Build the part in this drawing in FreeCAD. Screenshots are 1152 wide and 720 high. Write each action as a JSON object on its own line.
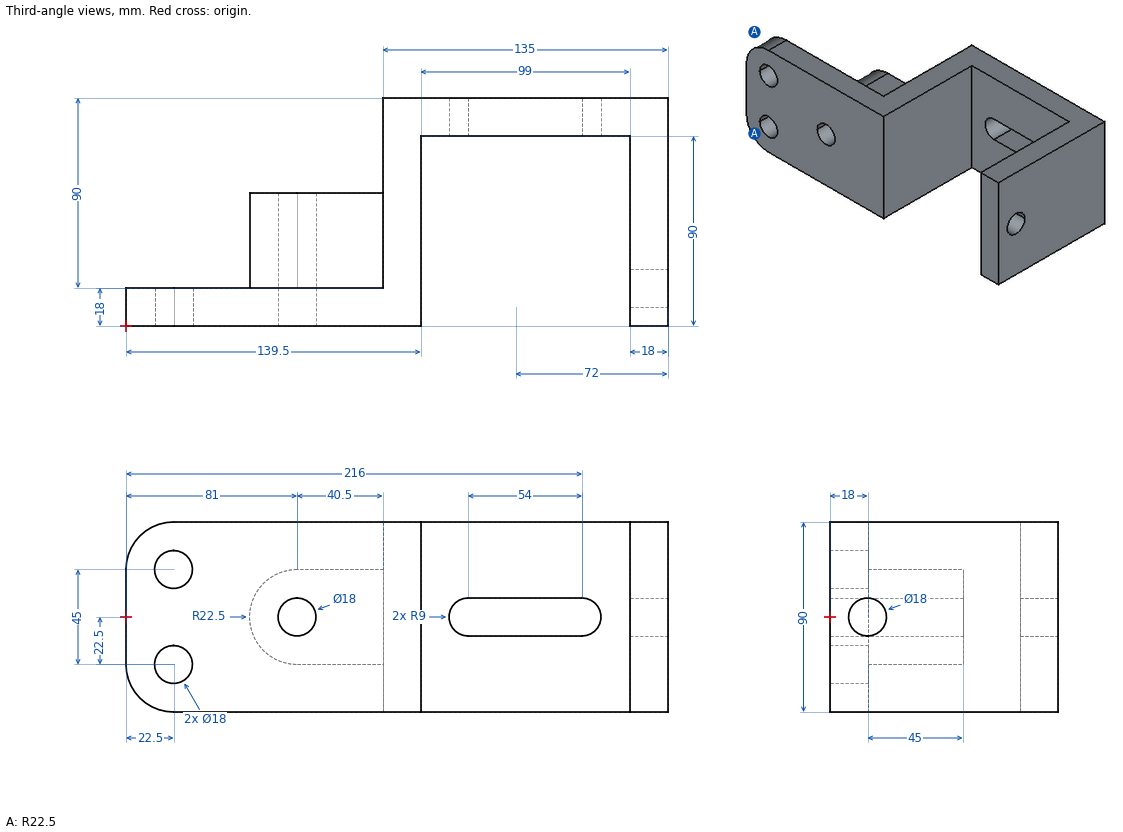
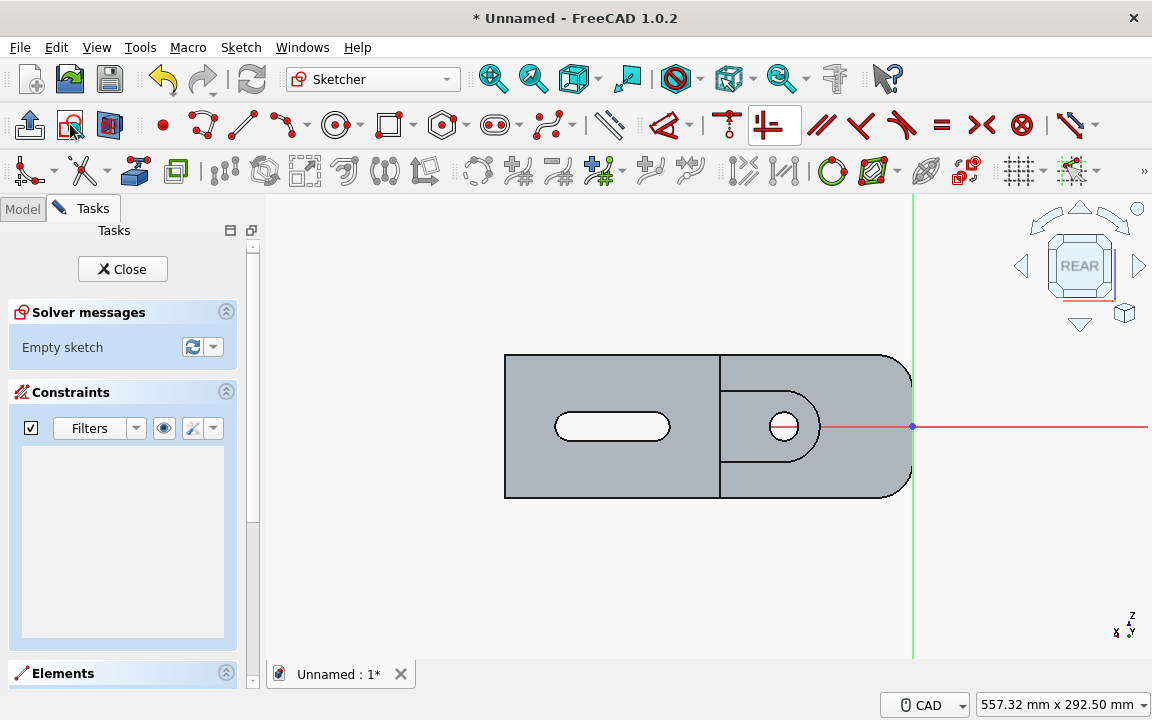
{"action": "left_click", "coordinate": [110, 126]}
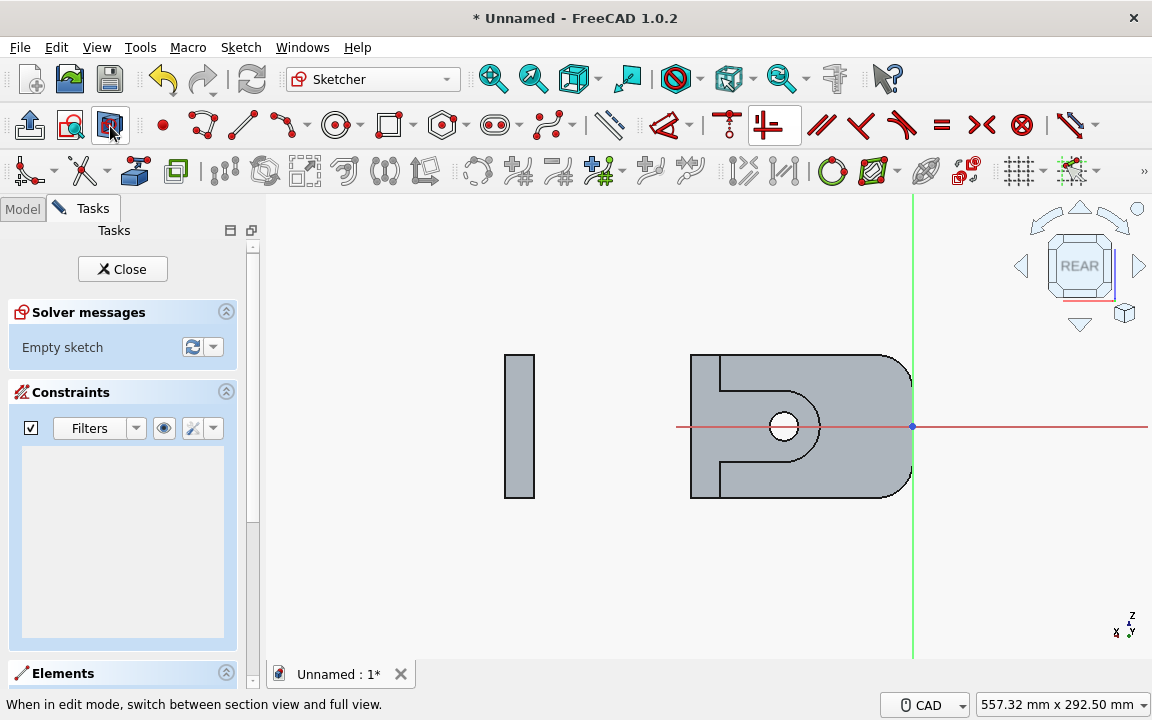
{"action": "scroll", "coordinate": [987, 426], "scroll_direction": "up", "scroll_amount": 5}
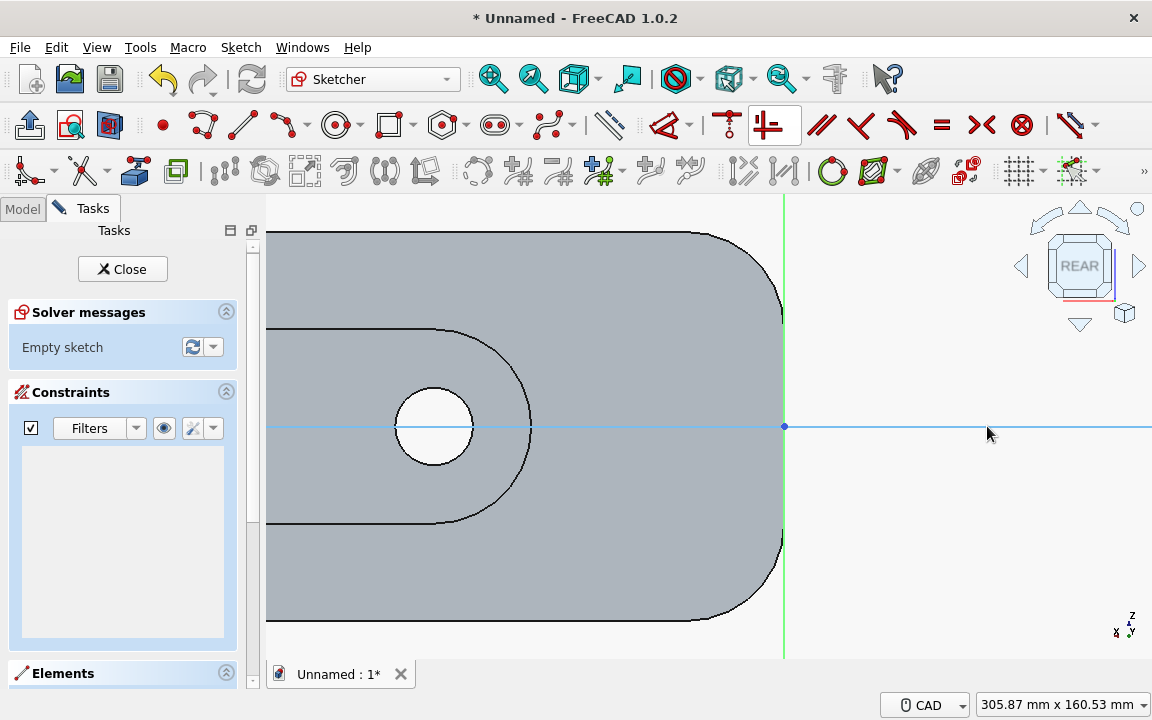
{"action": "left_click", "coordinate": [336, 126]}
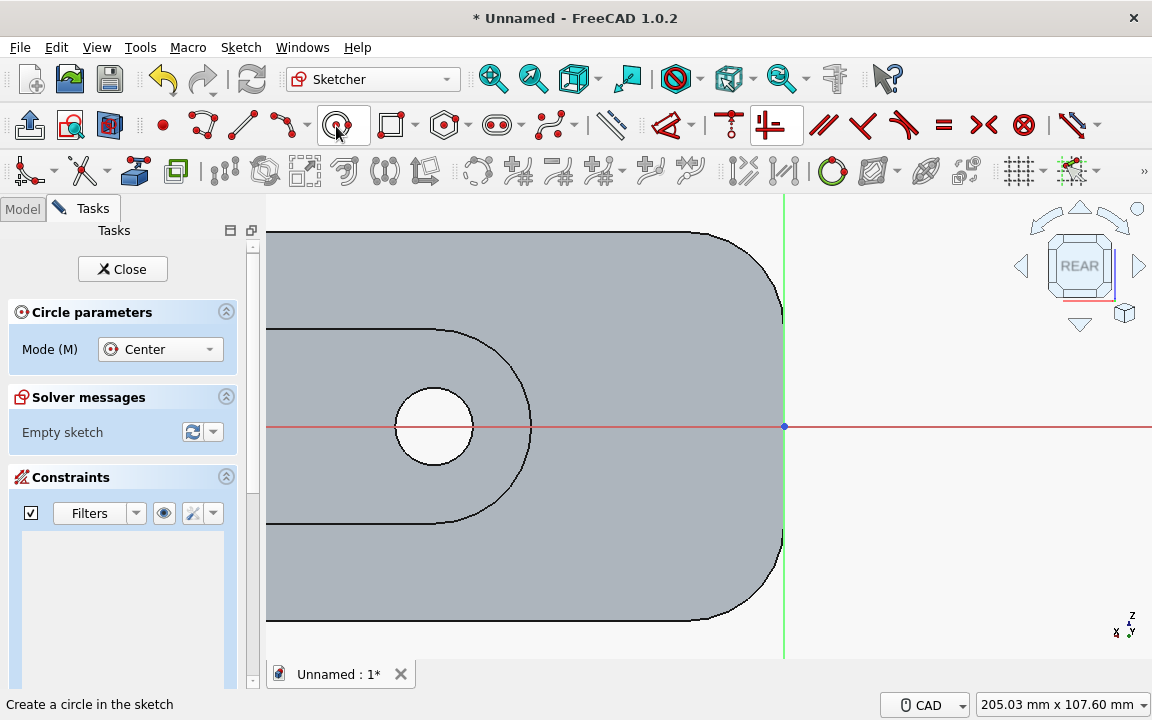
{"action": "left_click", "coordinate": [687, 524]}
{"action": "mouse_move", "coordinate": [714, 496]}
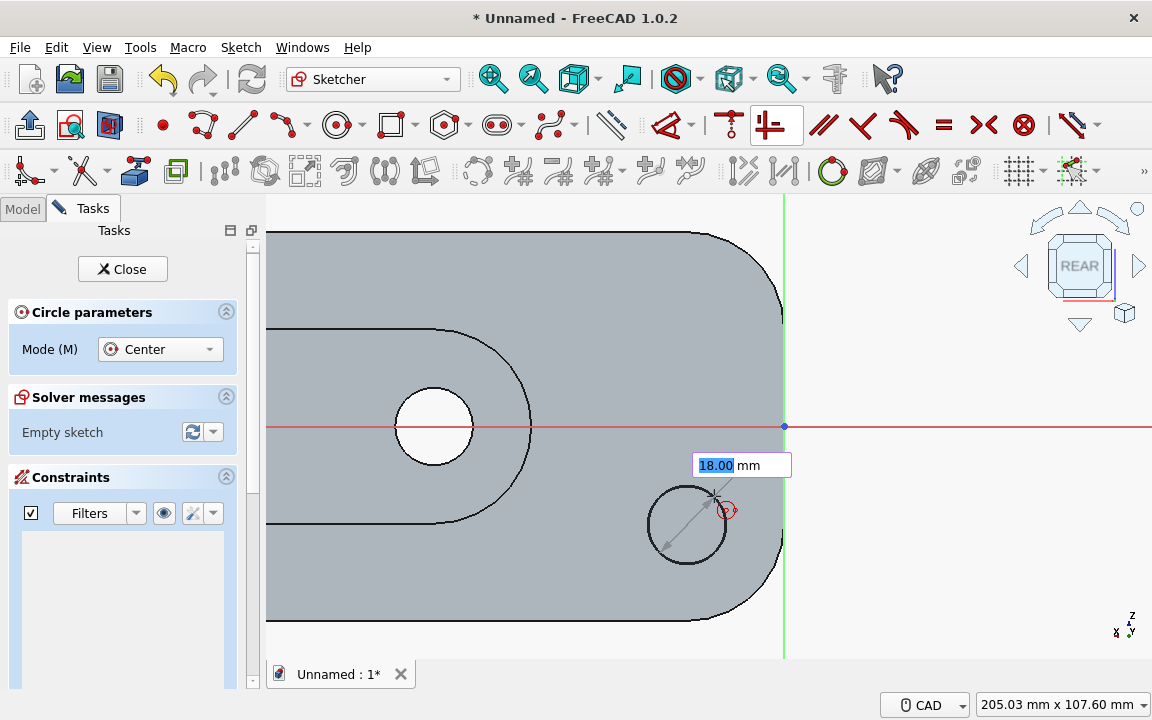
{"action": "type", "text": "18"}
{"action": "key", "text": "Return"}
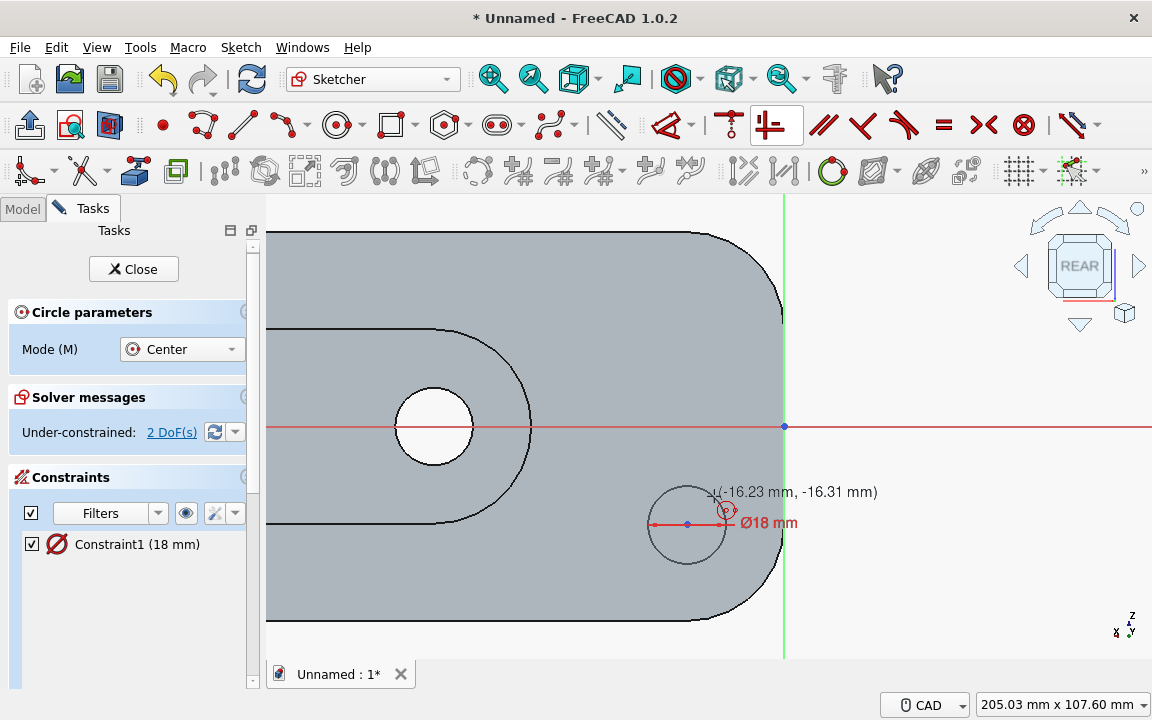
{"action": "left_click", "coordinate": [687, 329]}
{"action": "mouse_move", "coordinate": [714, 302]}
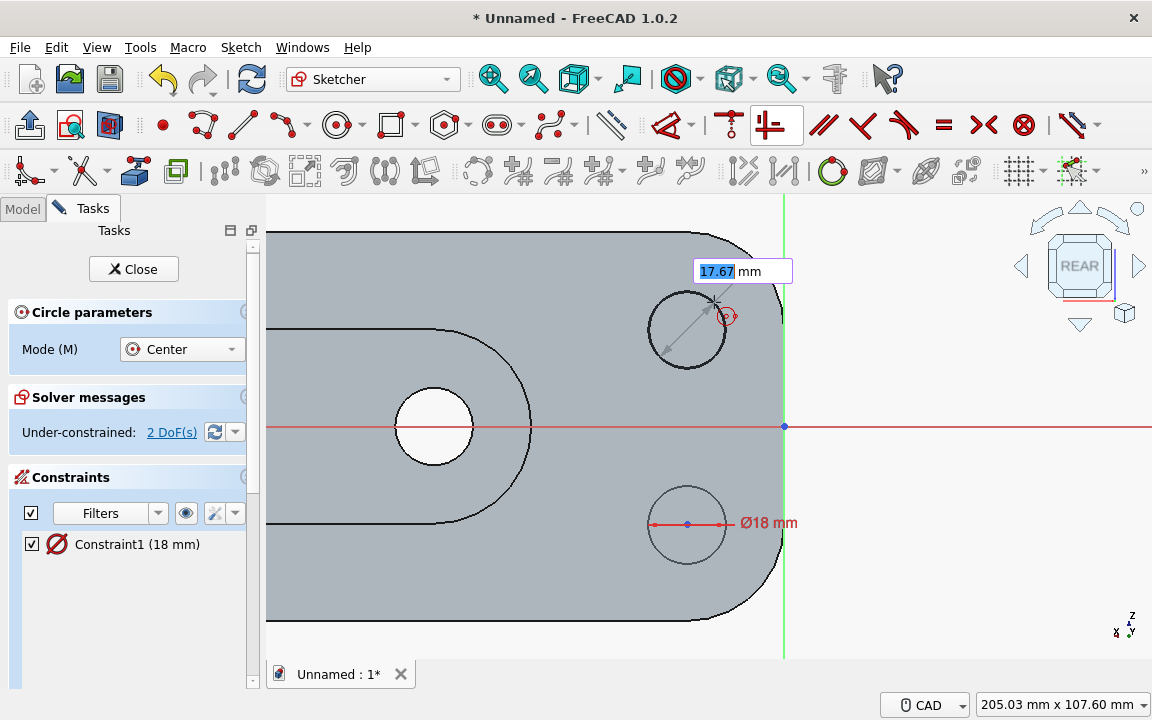
{"action": "type", "text": "18"}
{"action": "key", "text": "Return"}
{"action": "key", "text": "Escape"}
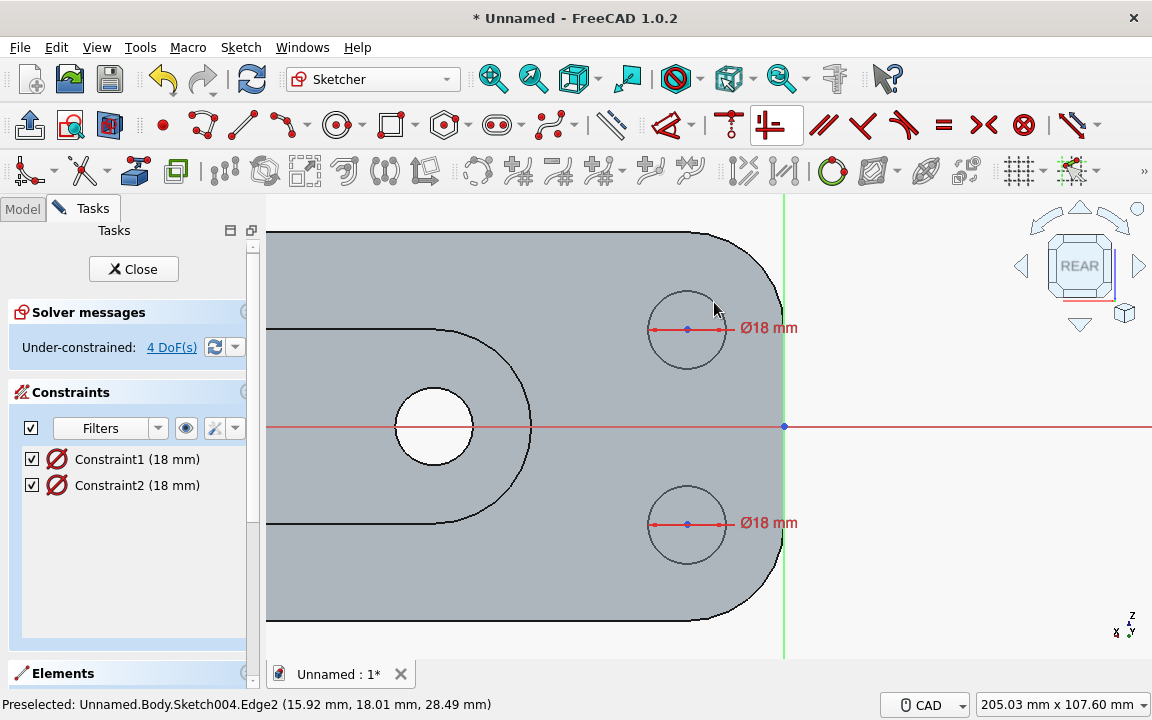
{"action": "left_click", "coordinate": [687, 525]}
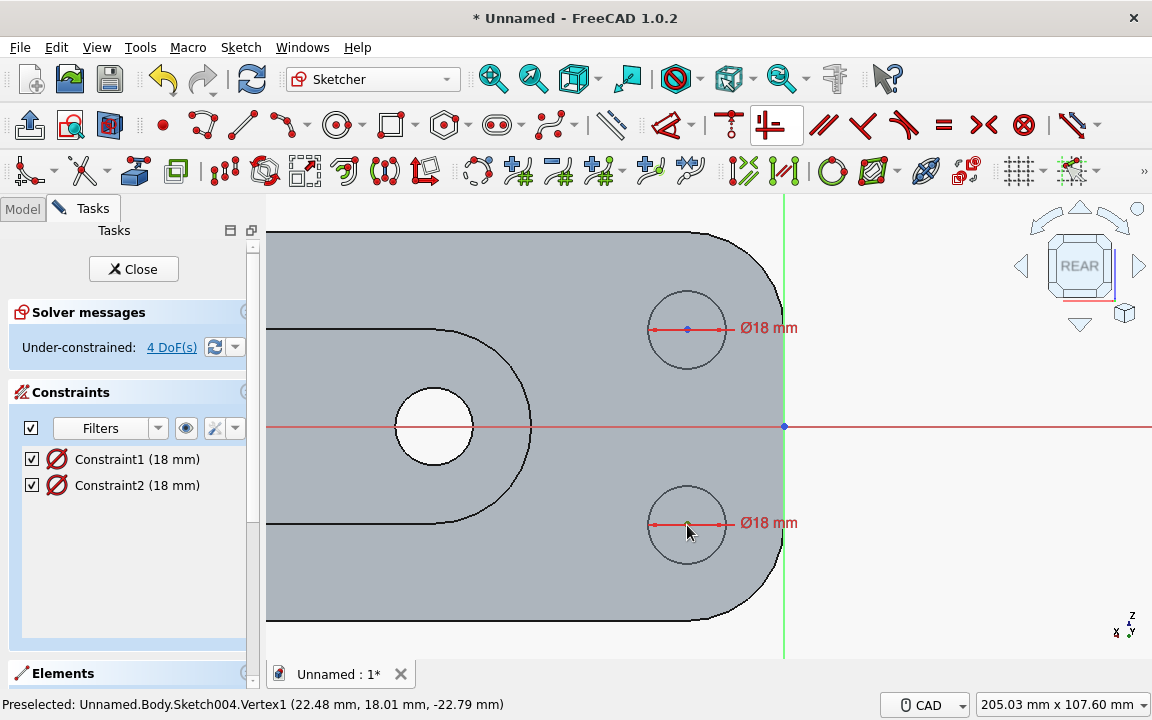
{"action": "left_click", "coordinate": [687, 330]}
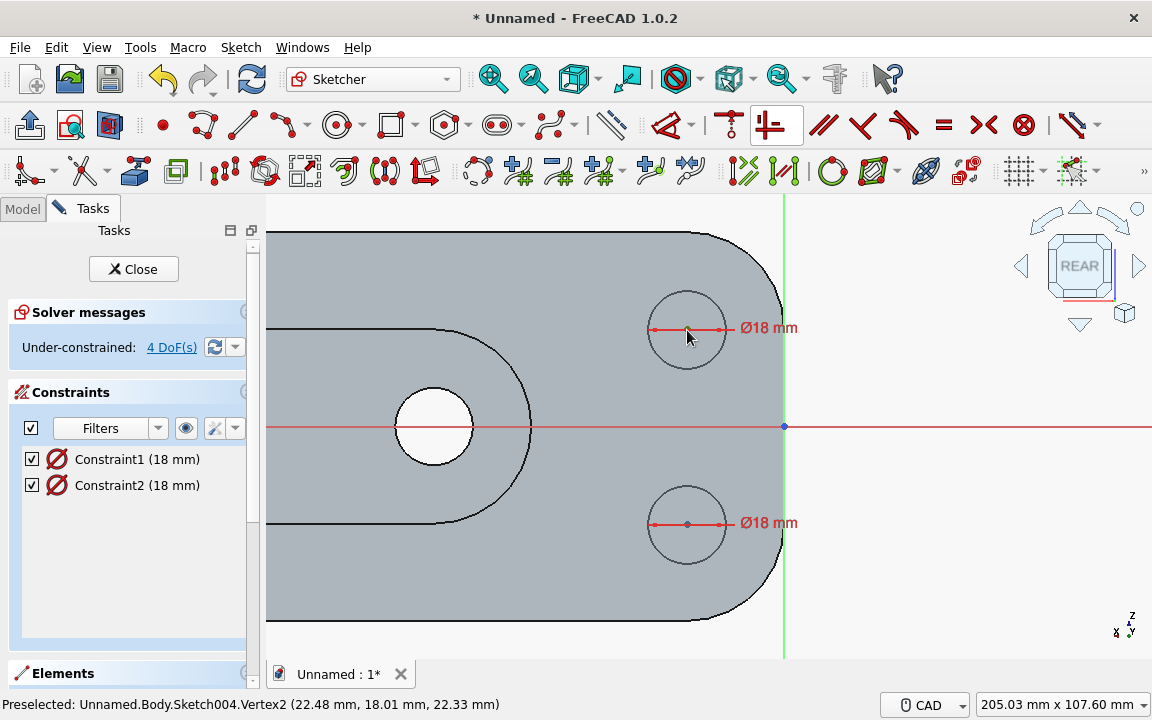
{"action": "key", "text": "v"}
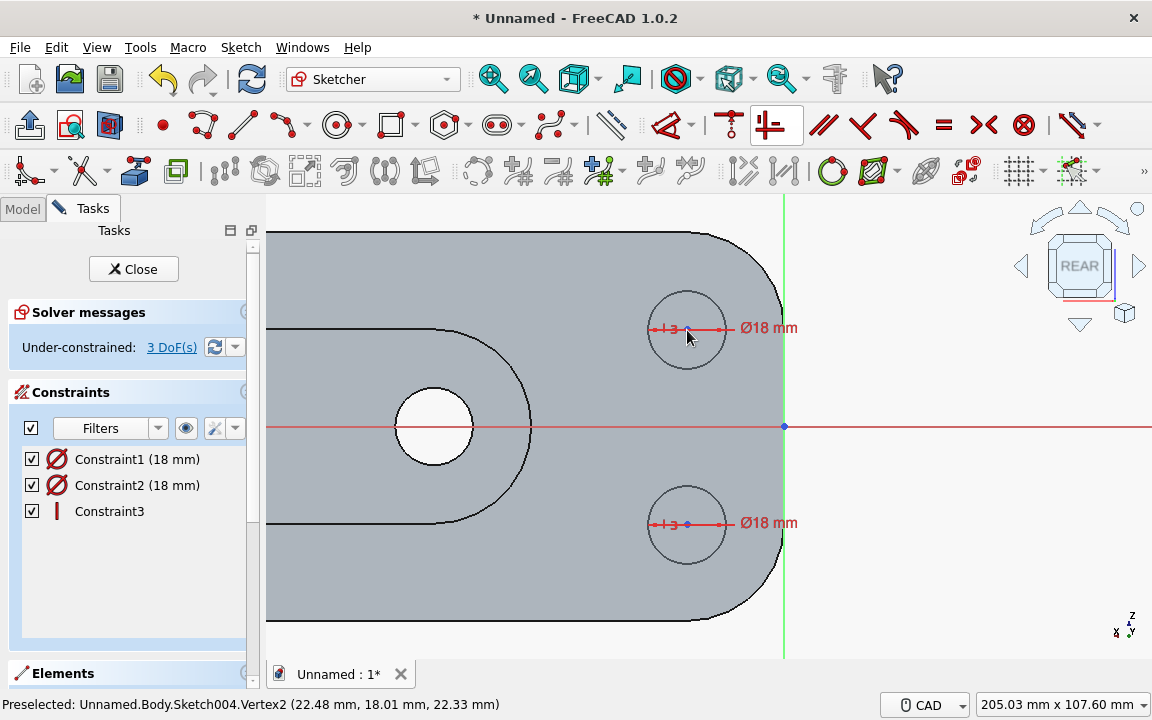
{"action": "key", "text": "d"}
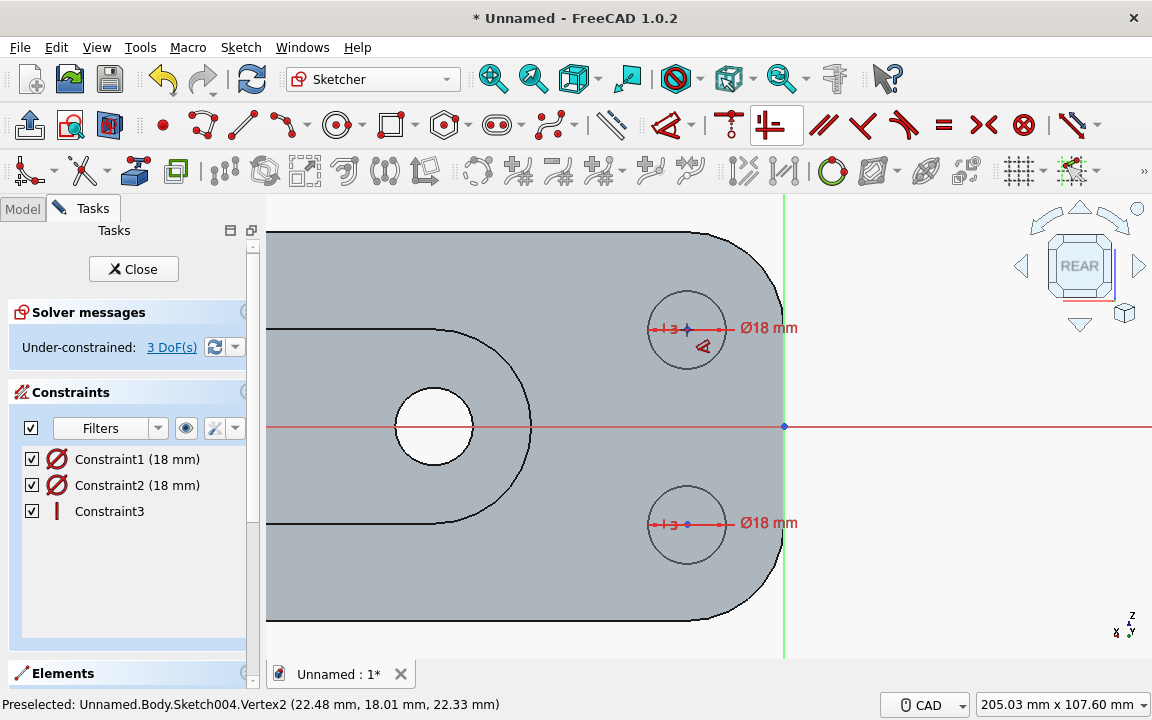
{"action": "left_click", "coordinate": [687, 525]}